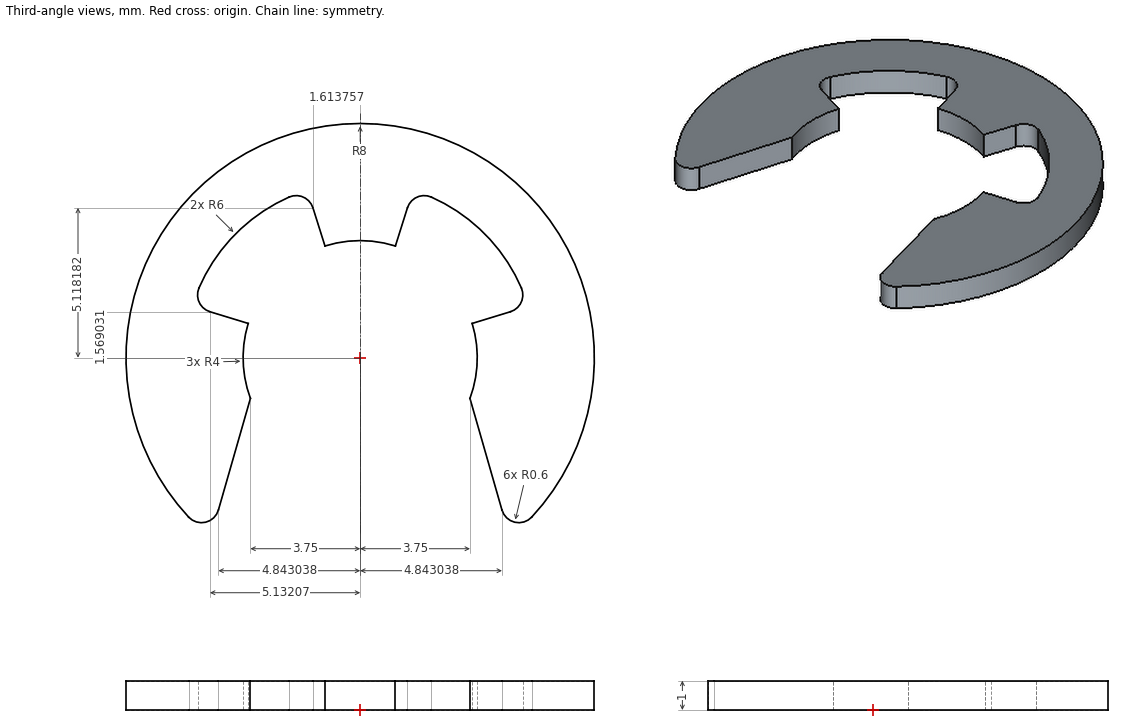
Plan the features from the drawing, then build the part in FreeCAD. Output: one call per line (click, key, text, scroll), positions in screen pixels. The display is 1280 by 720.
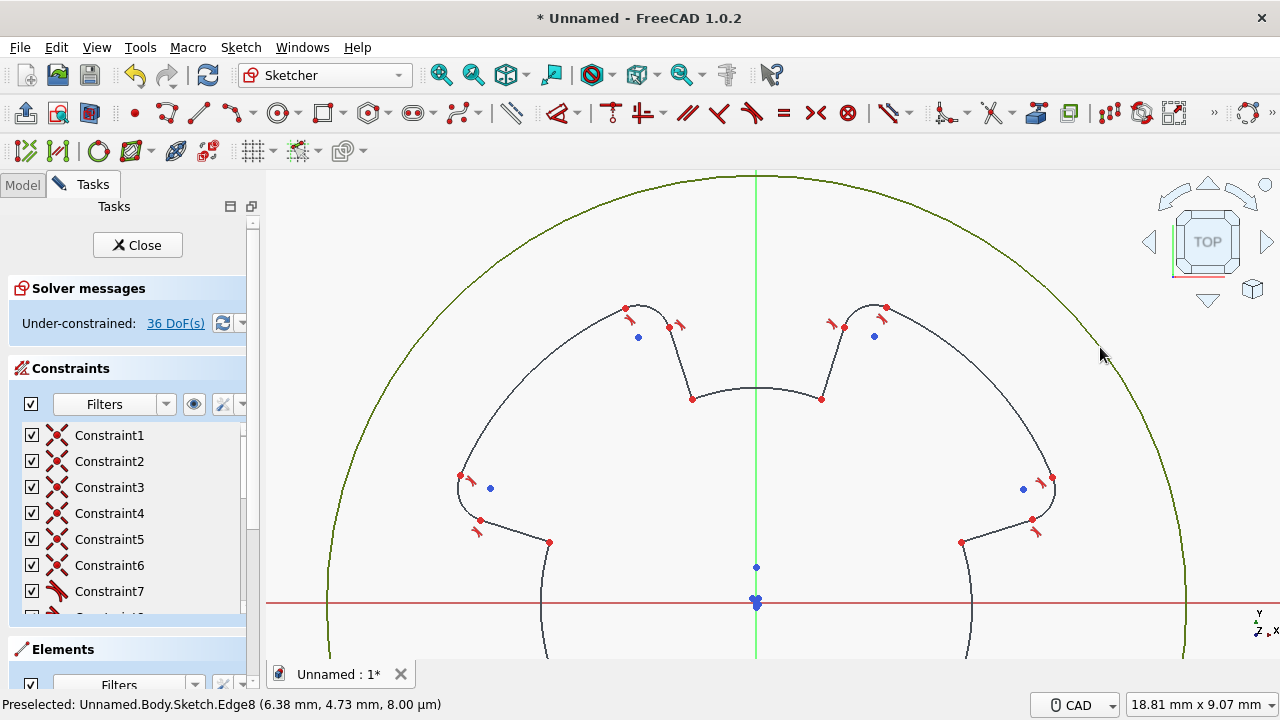
click(542, 583)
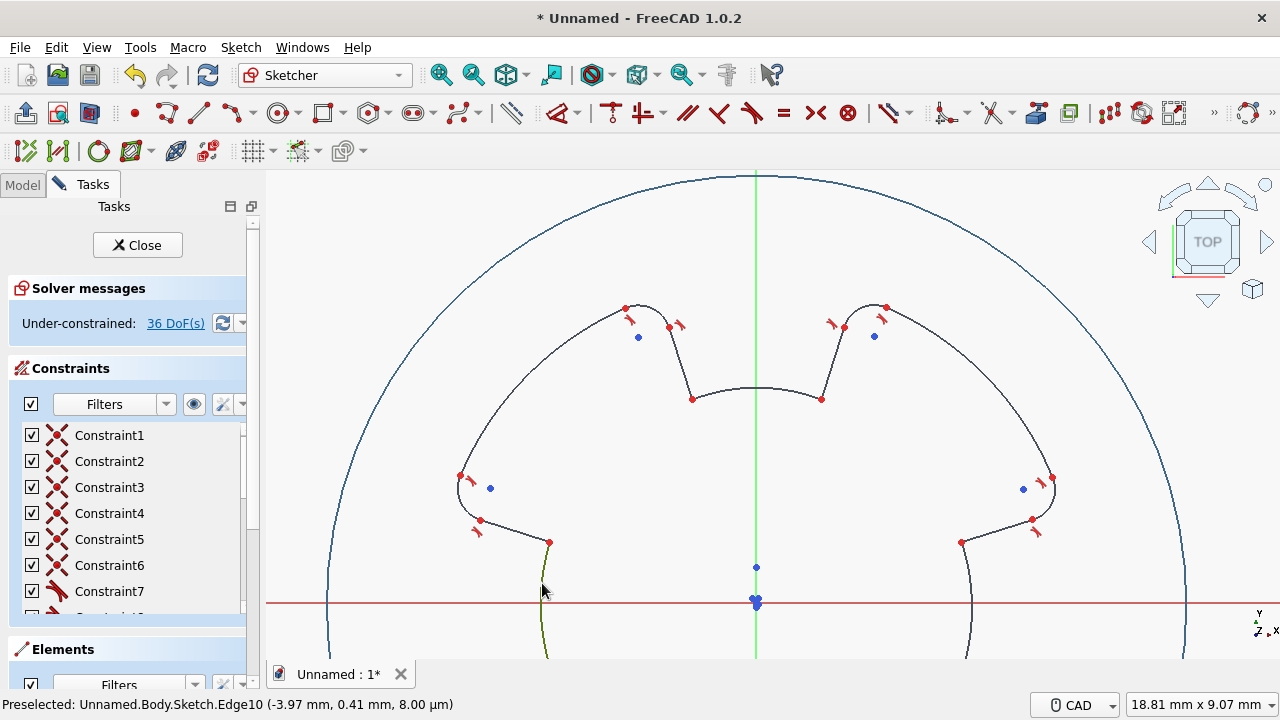
key(c)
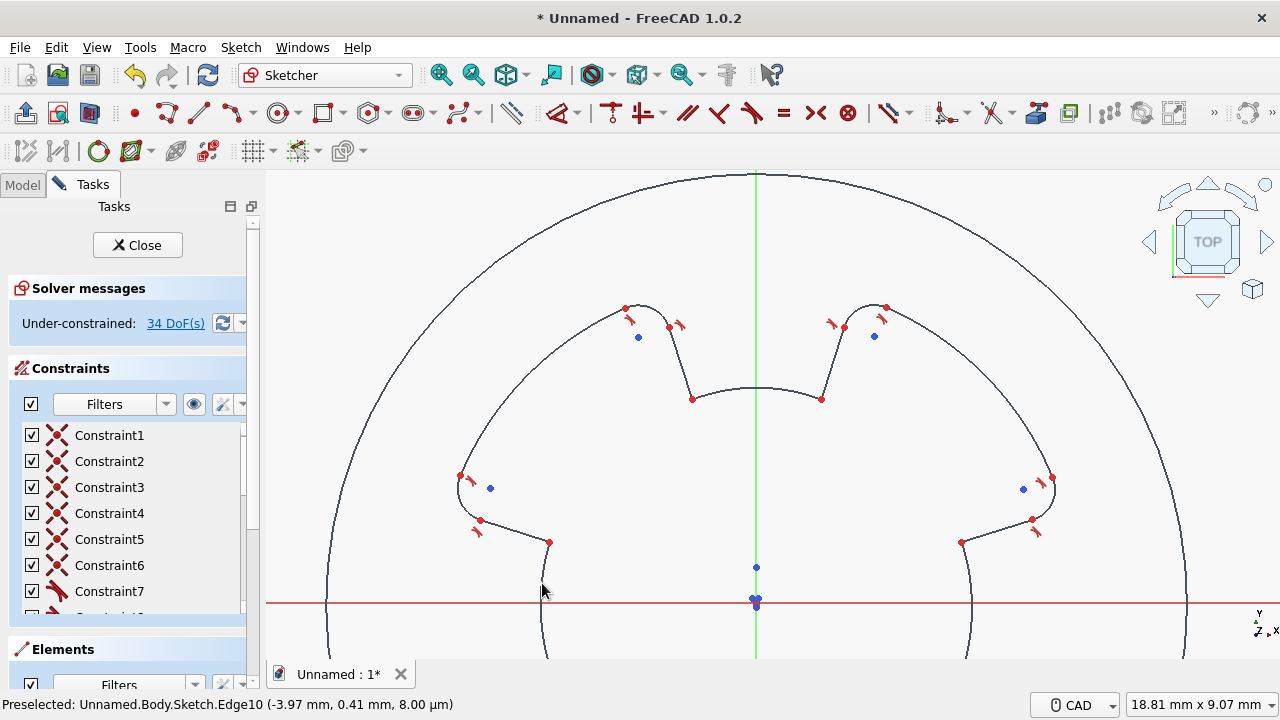
click(1101, 346)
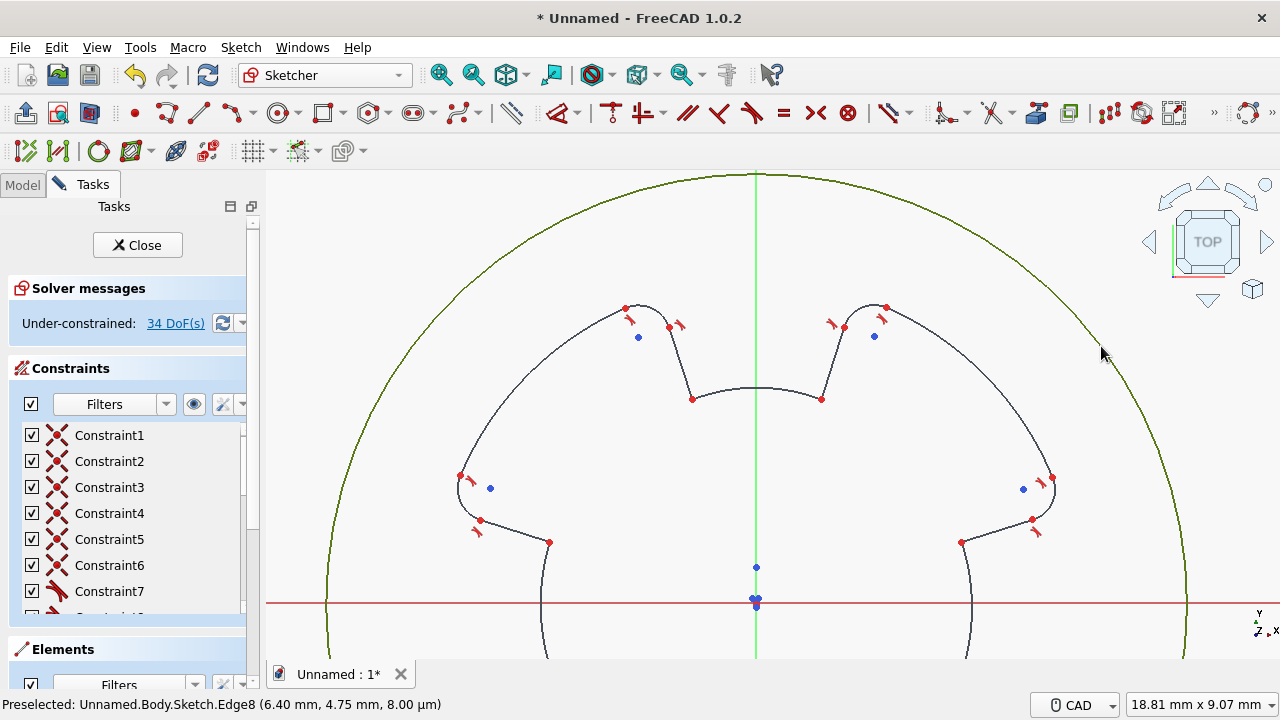
click(563, 345)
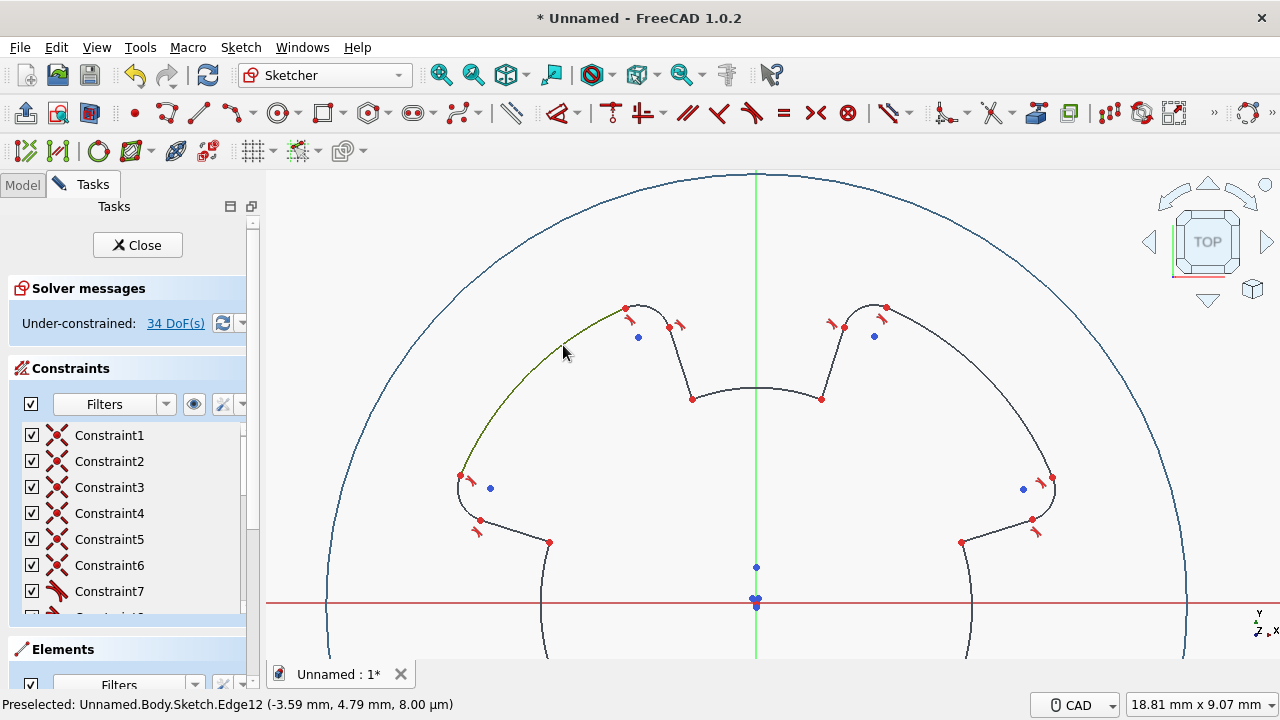
click(612, 114)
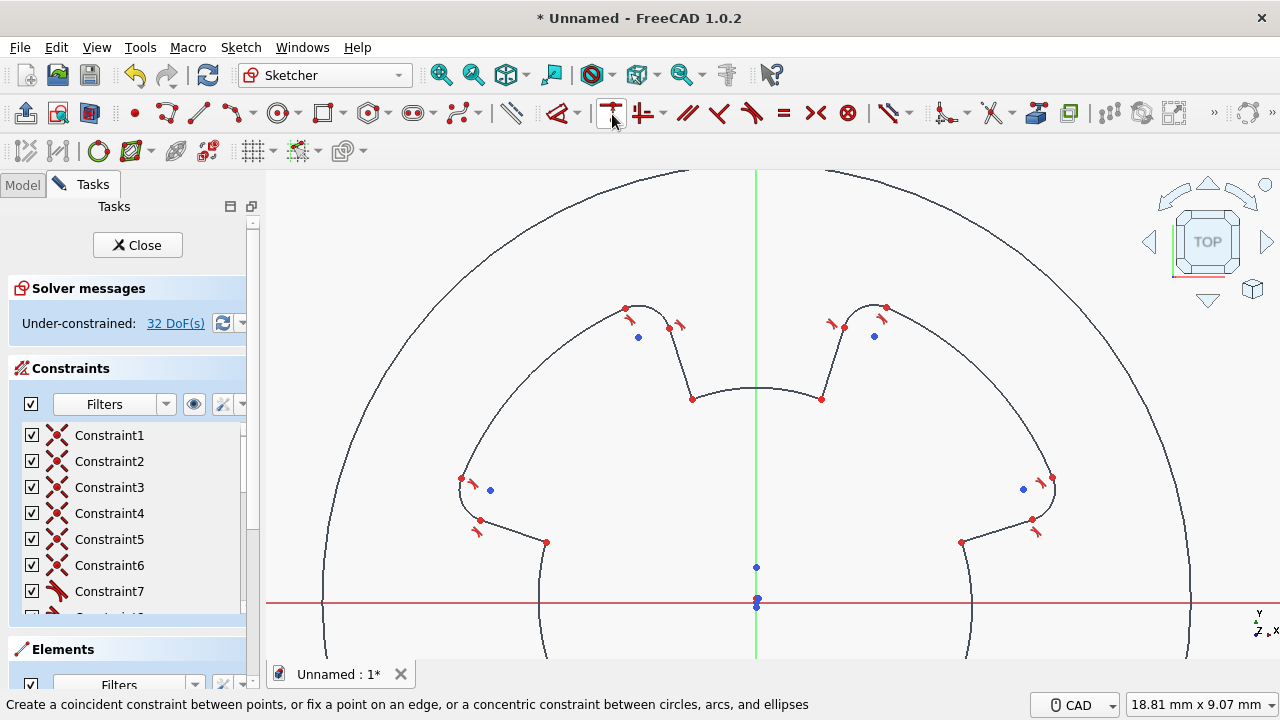
click(1105, 339)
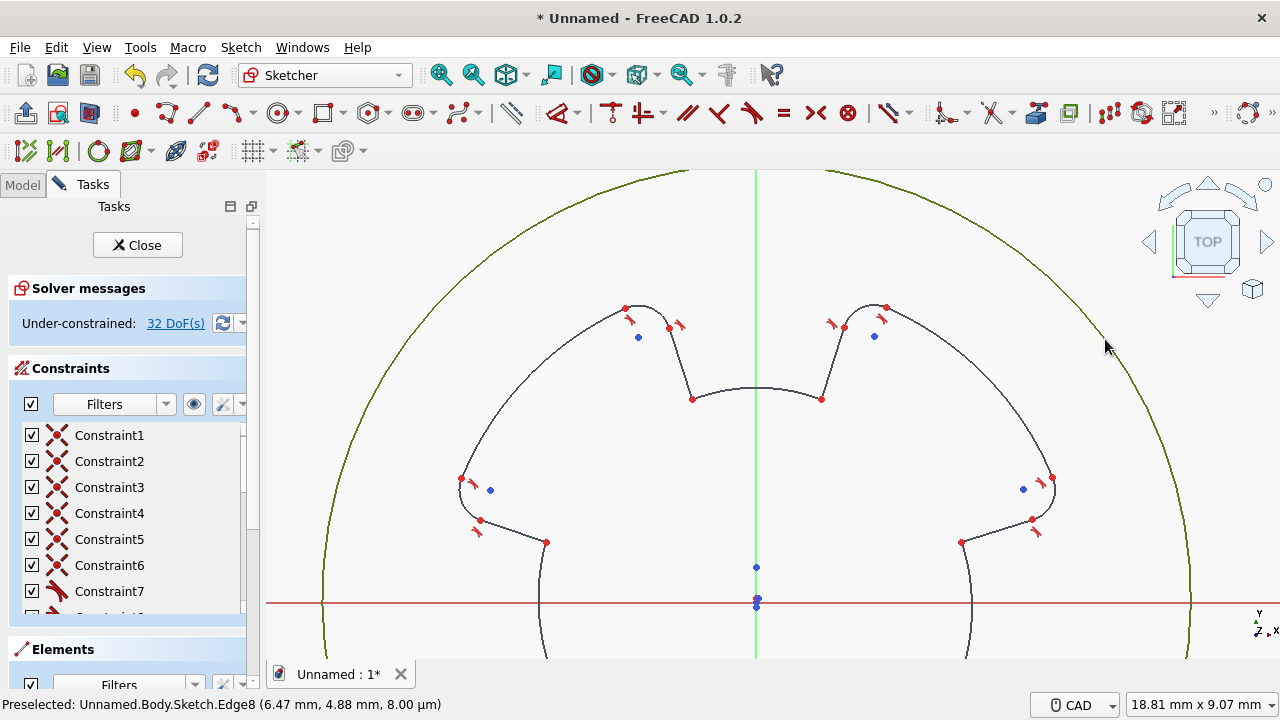
click(783, 390)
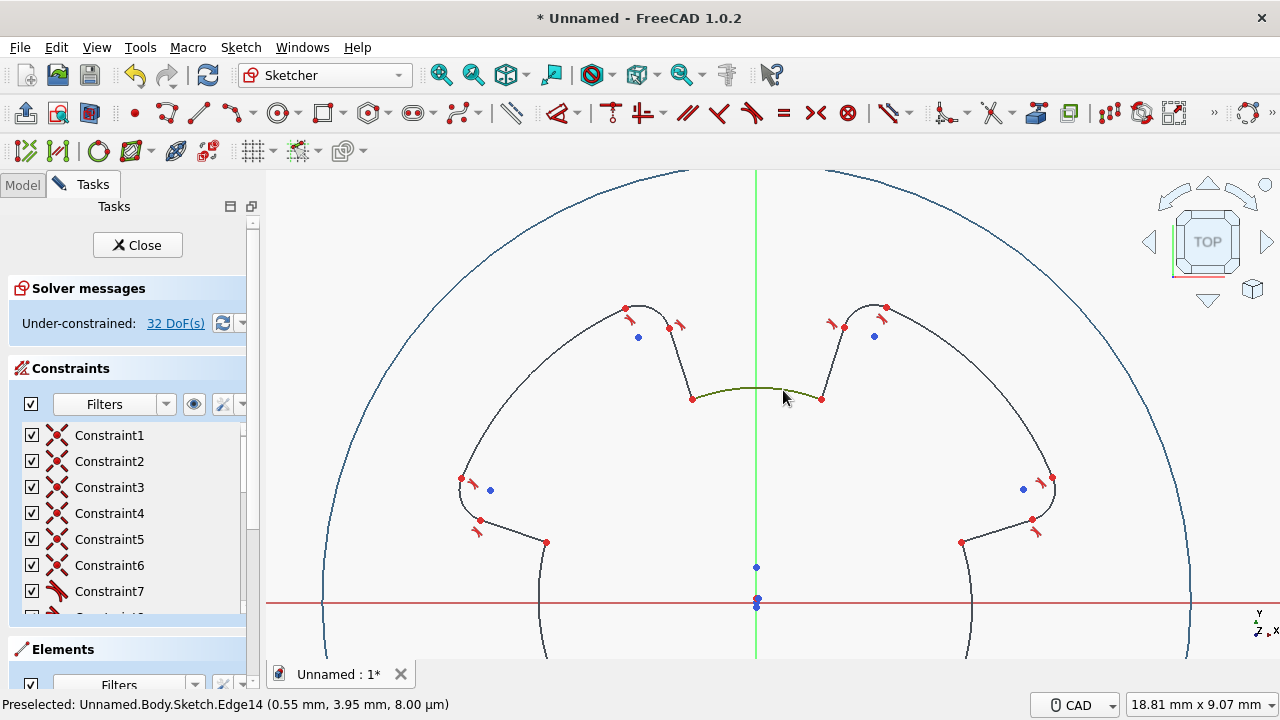
click(612, 114)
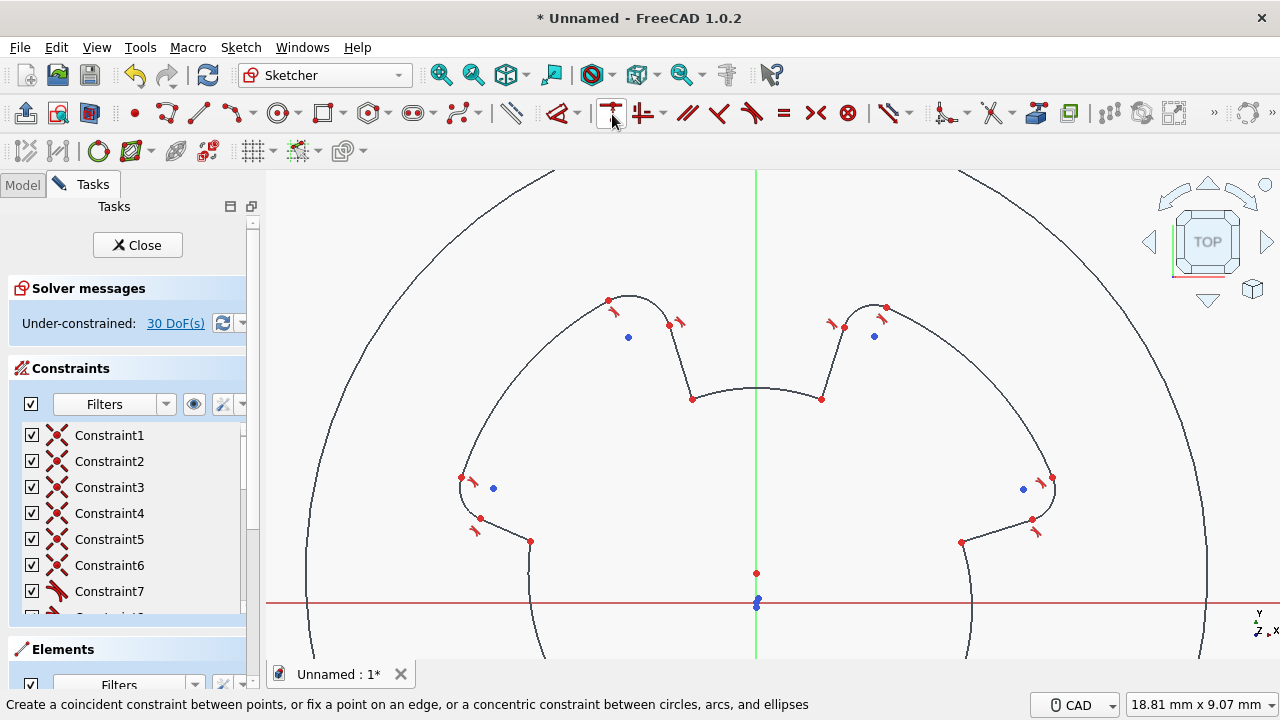
click(390, 310)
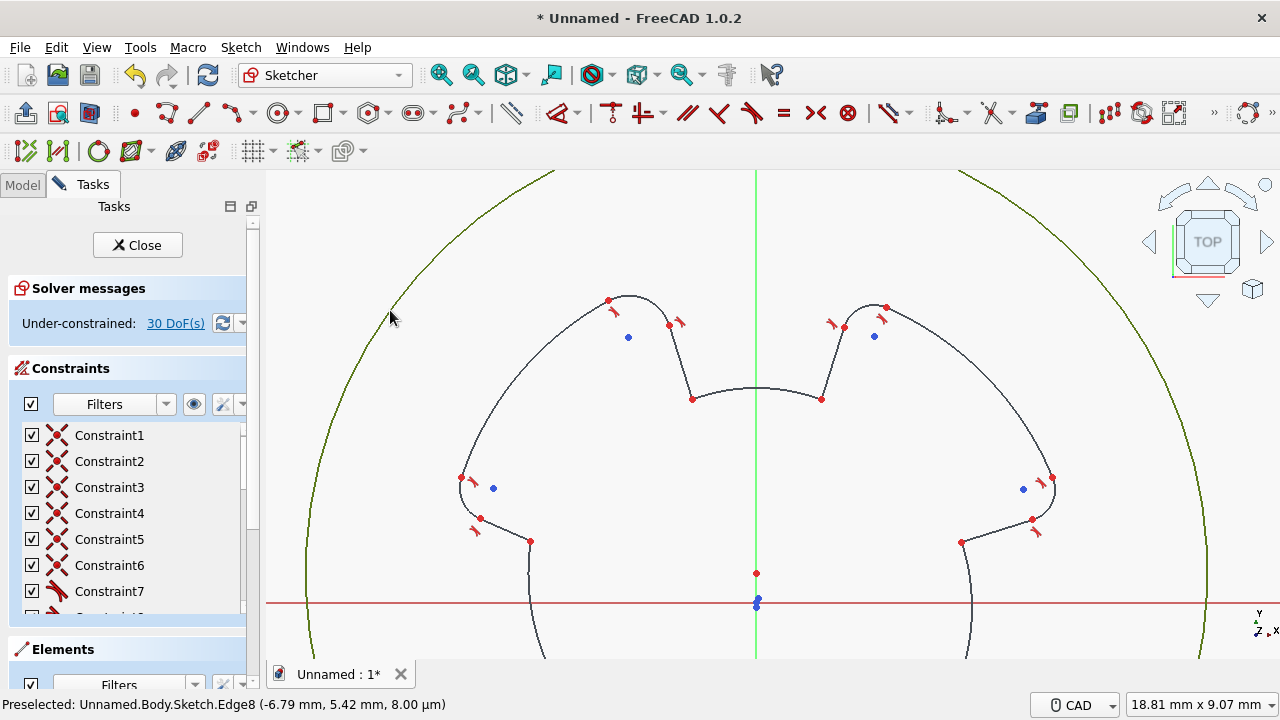
click(1017, 414)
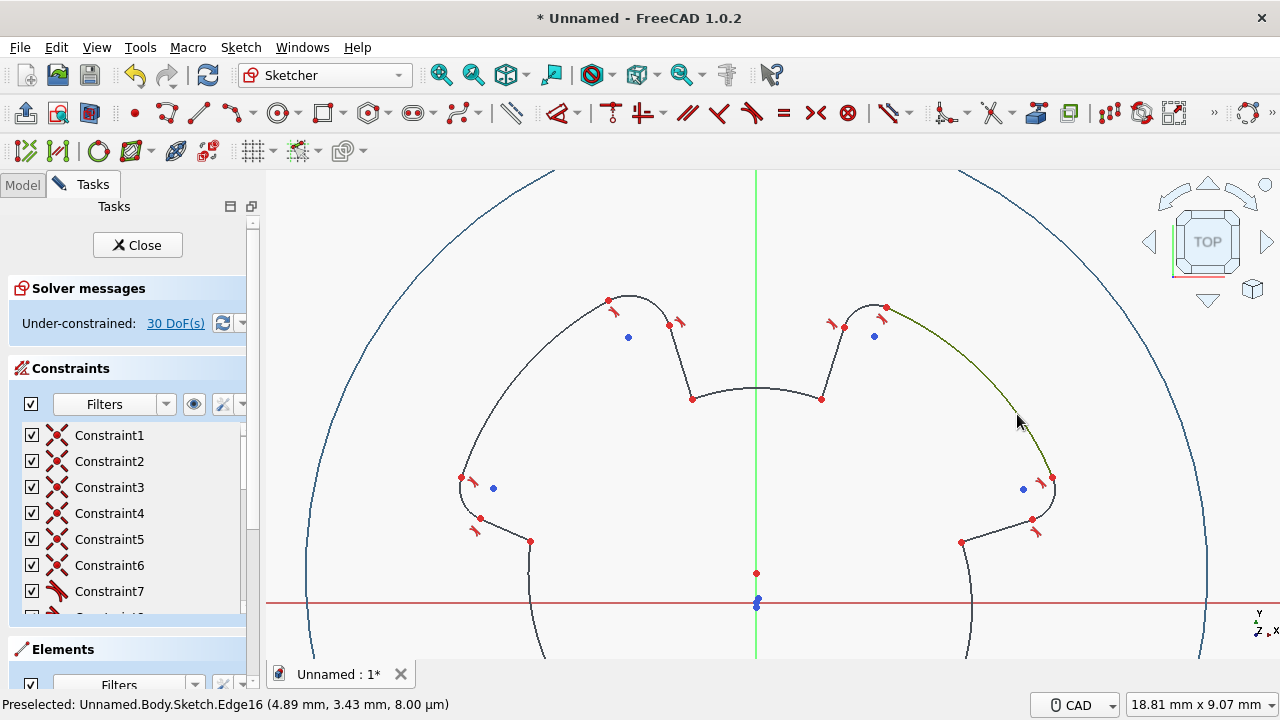
click(612, 114)